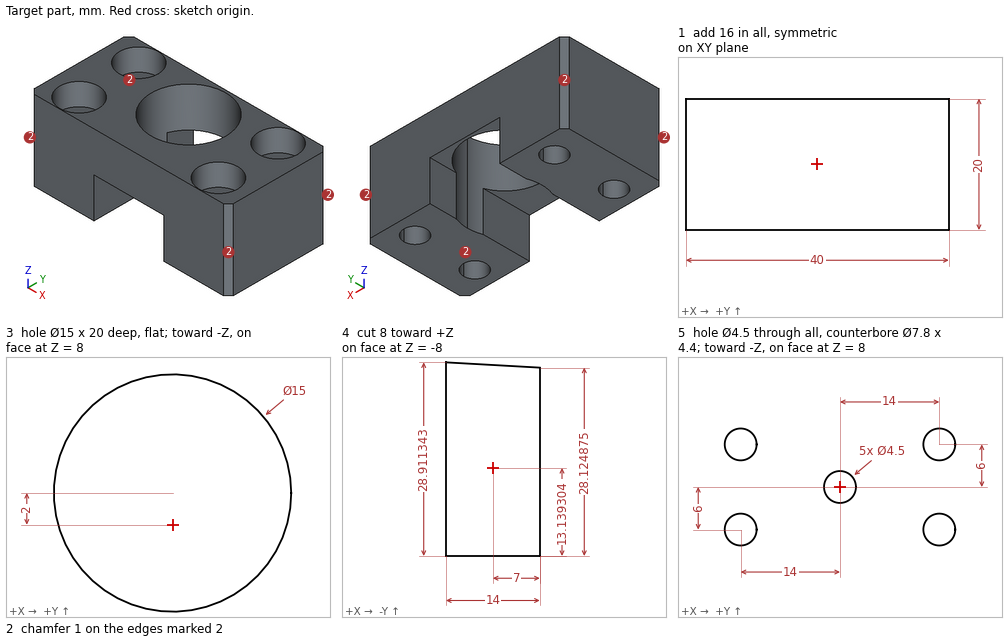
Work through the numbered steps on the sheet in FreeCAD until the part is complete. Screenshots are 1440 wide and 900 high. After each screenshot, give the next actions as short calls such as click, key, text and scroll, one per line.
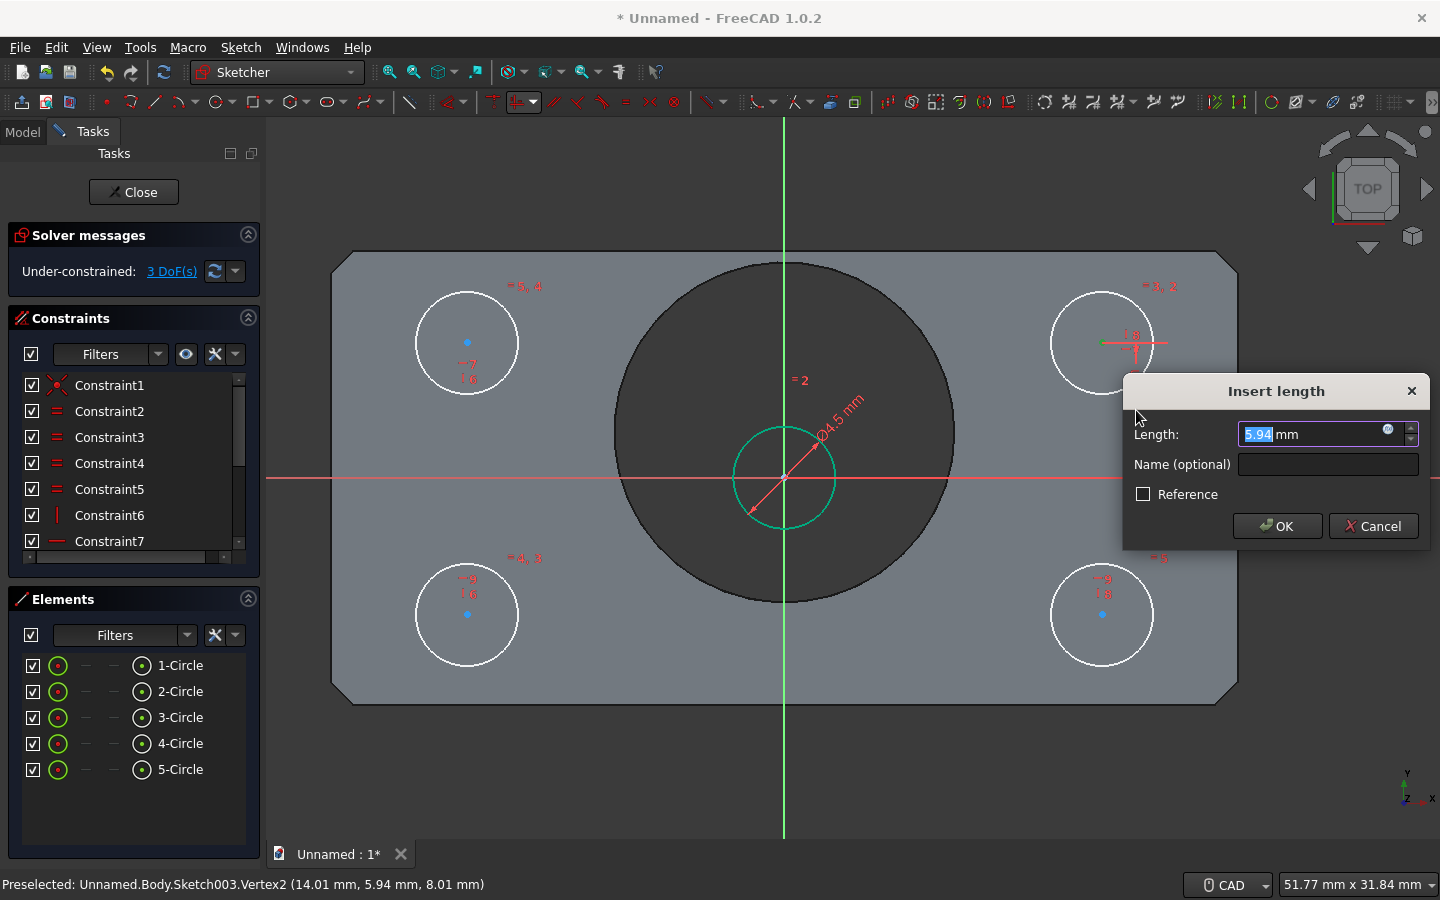
text(6)
key(Return)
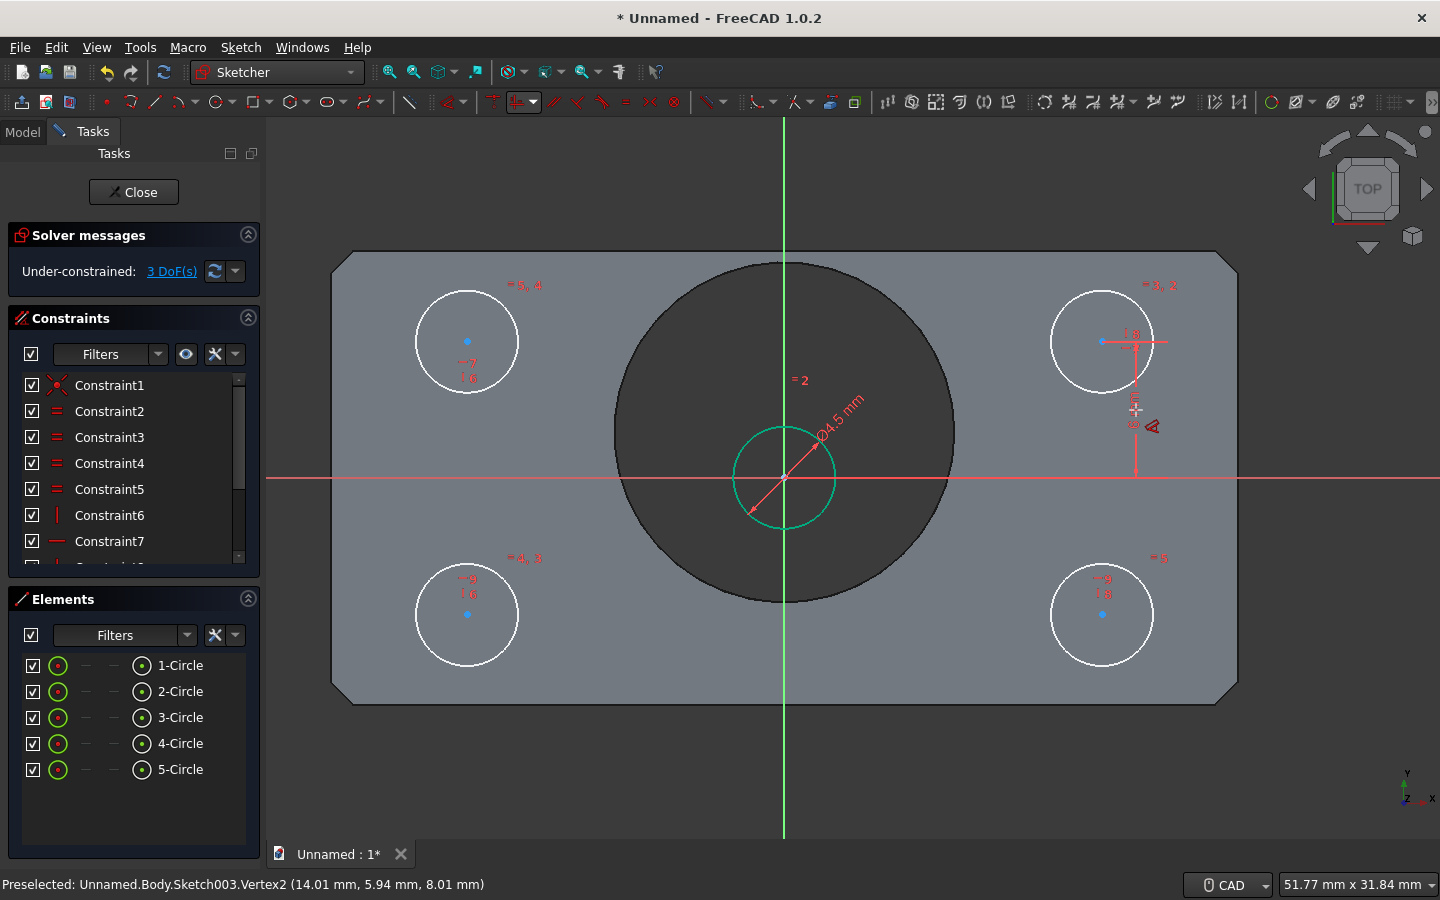
click(467, 615)
click(433, 546)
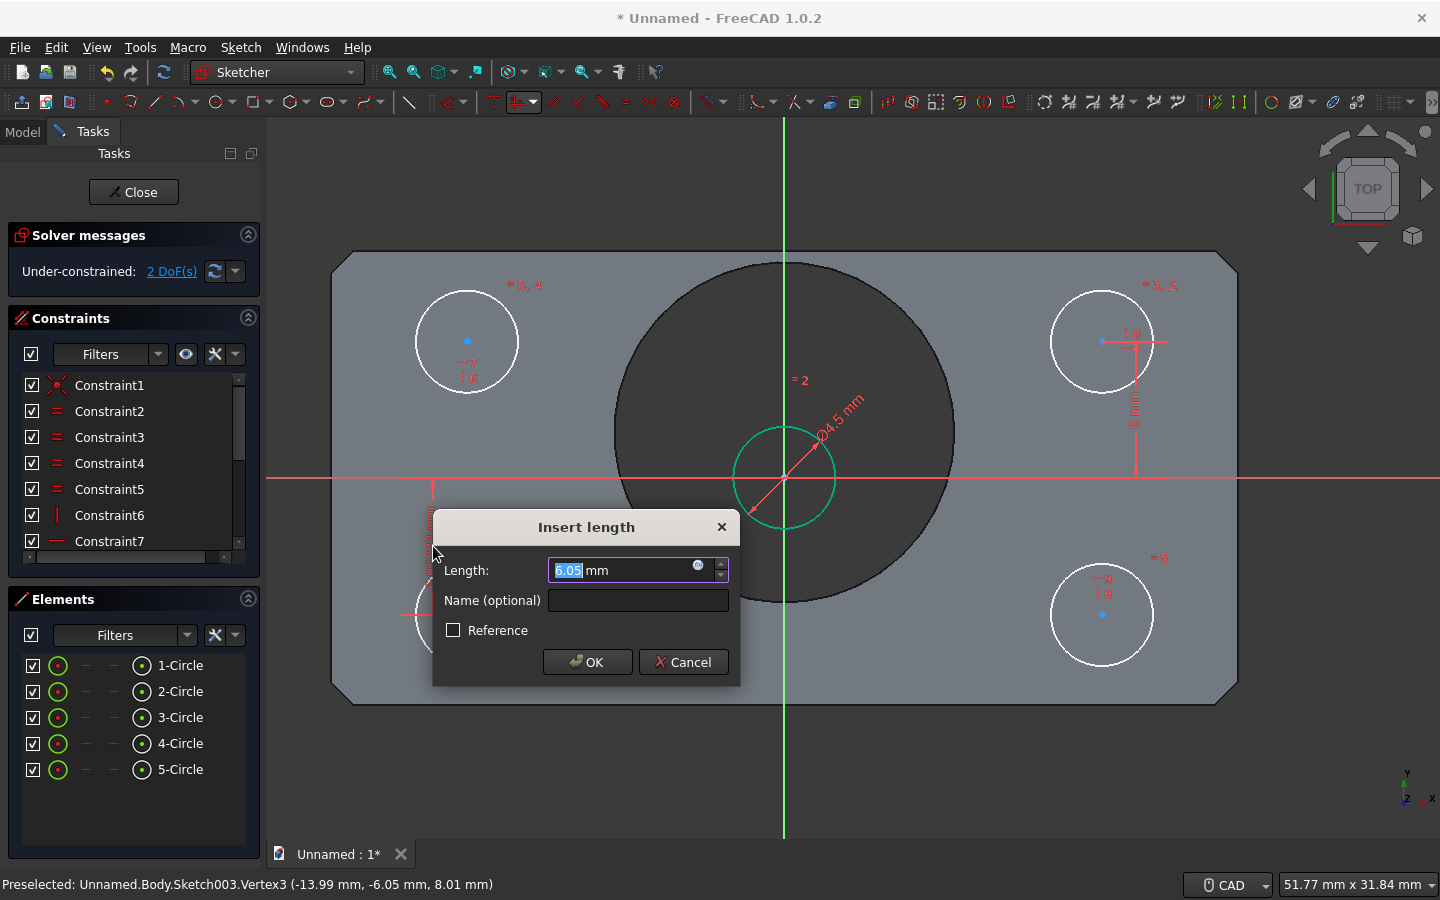
text(6)
key(Return)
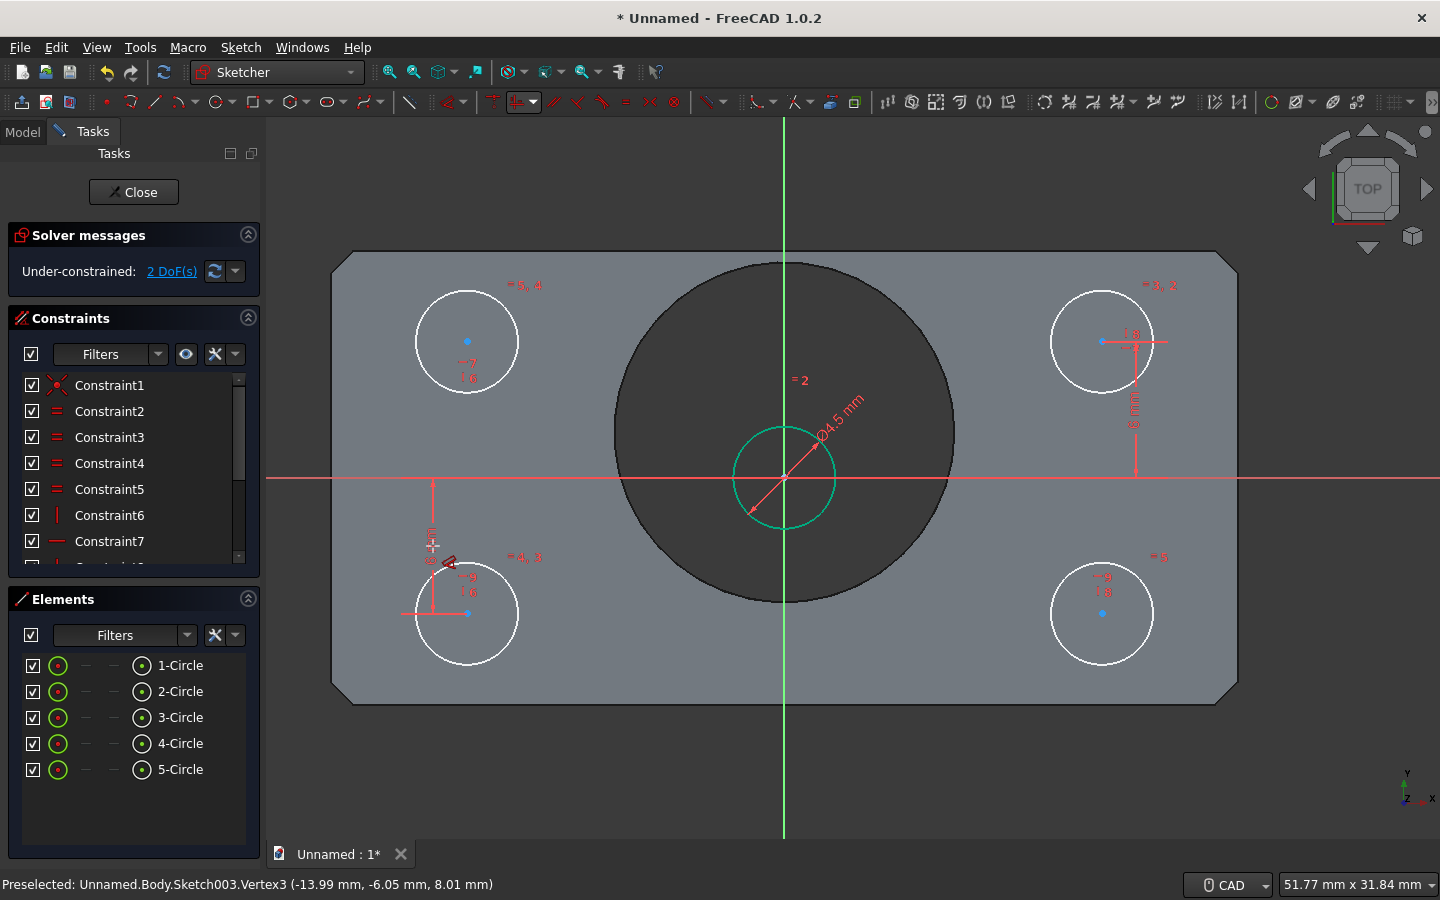
click(1102, 342)
click(943, 308)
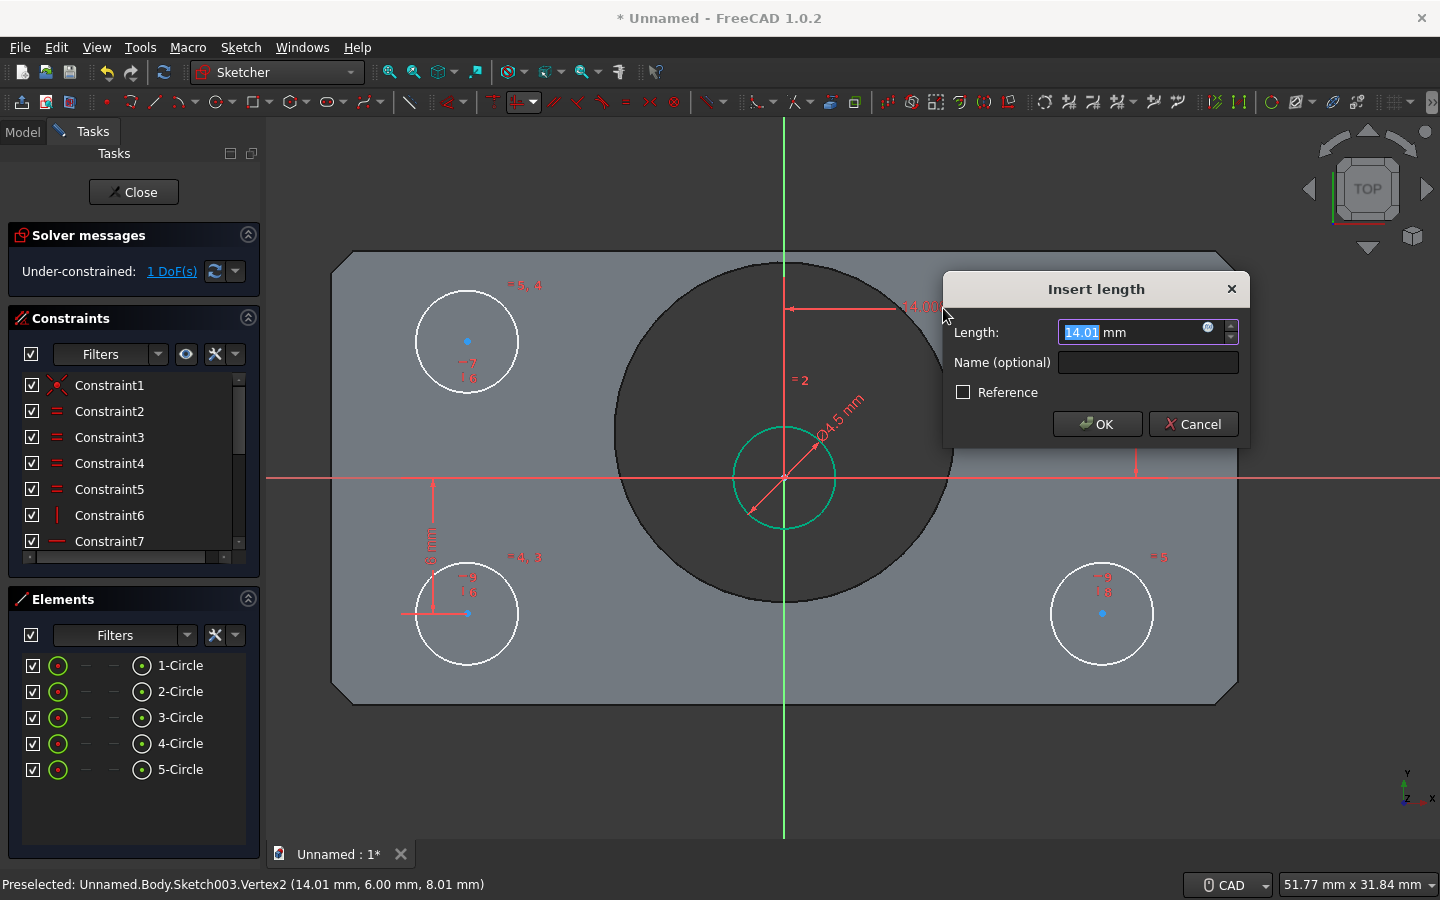
text(14)
key(Return)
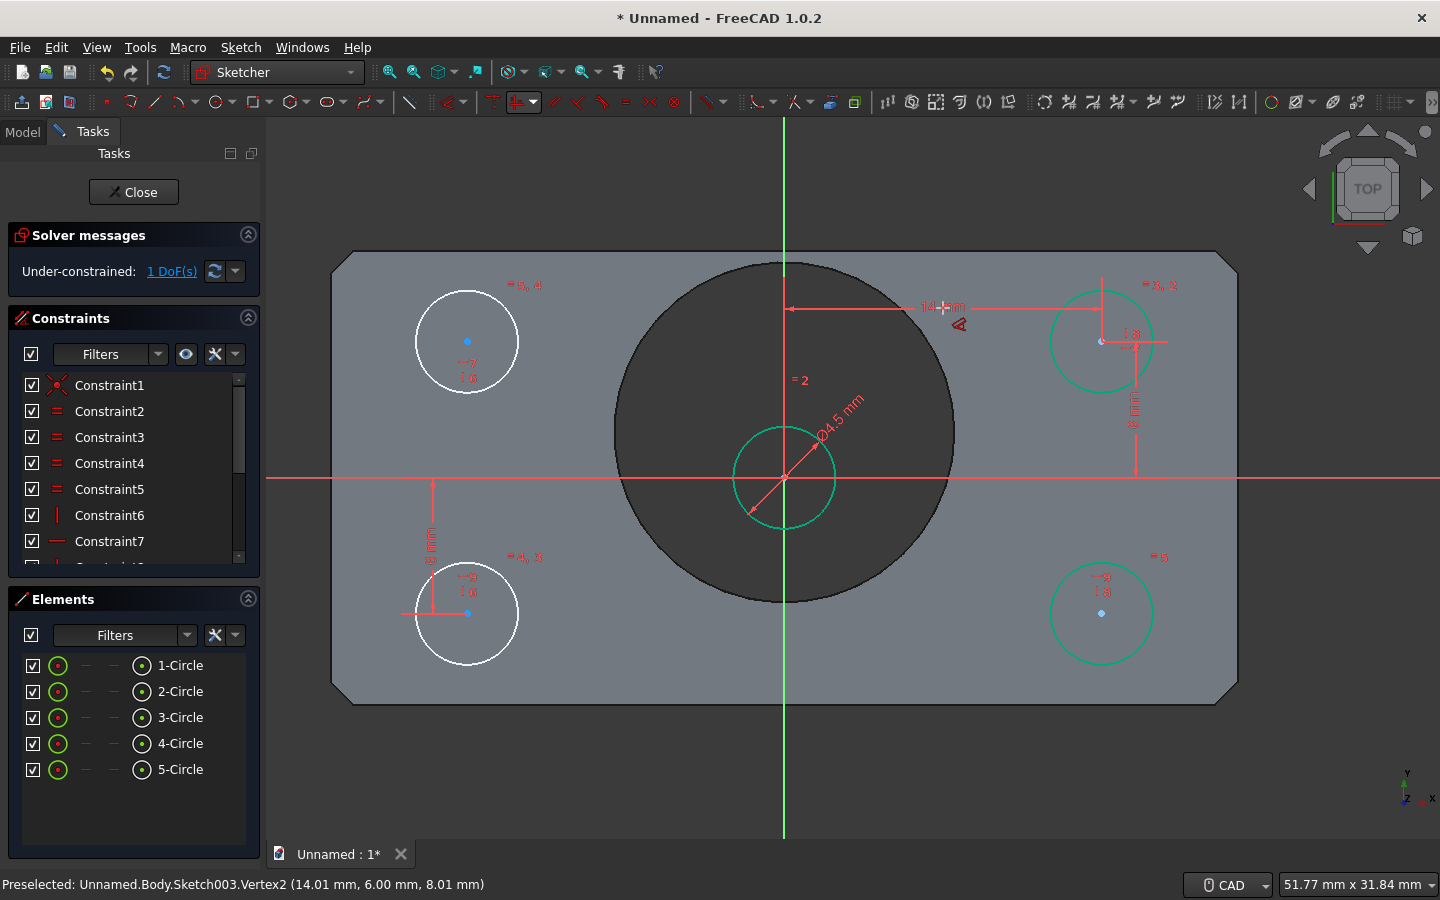
click(467, 614)
click(626, 648)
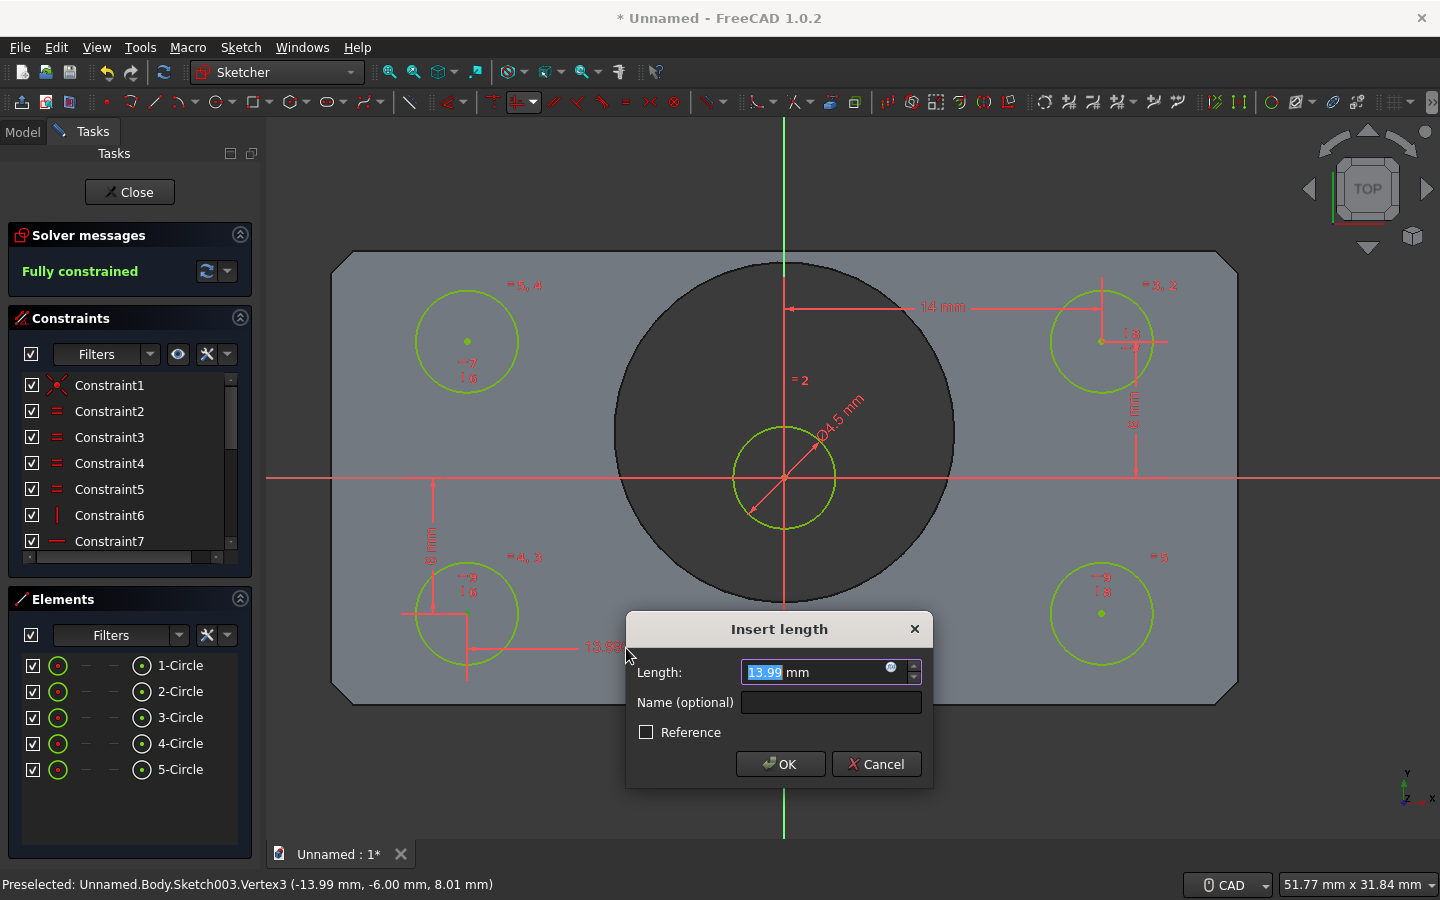
text(14)
key(Return)
key(Escape)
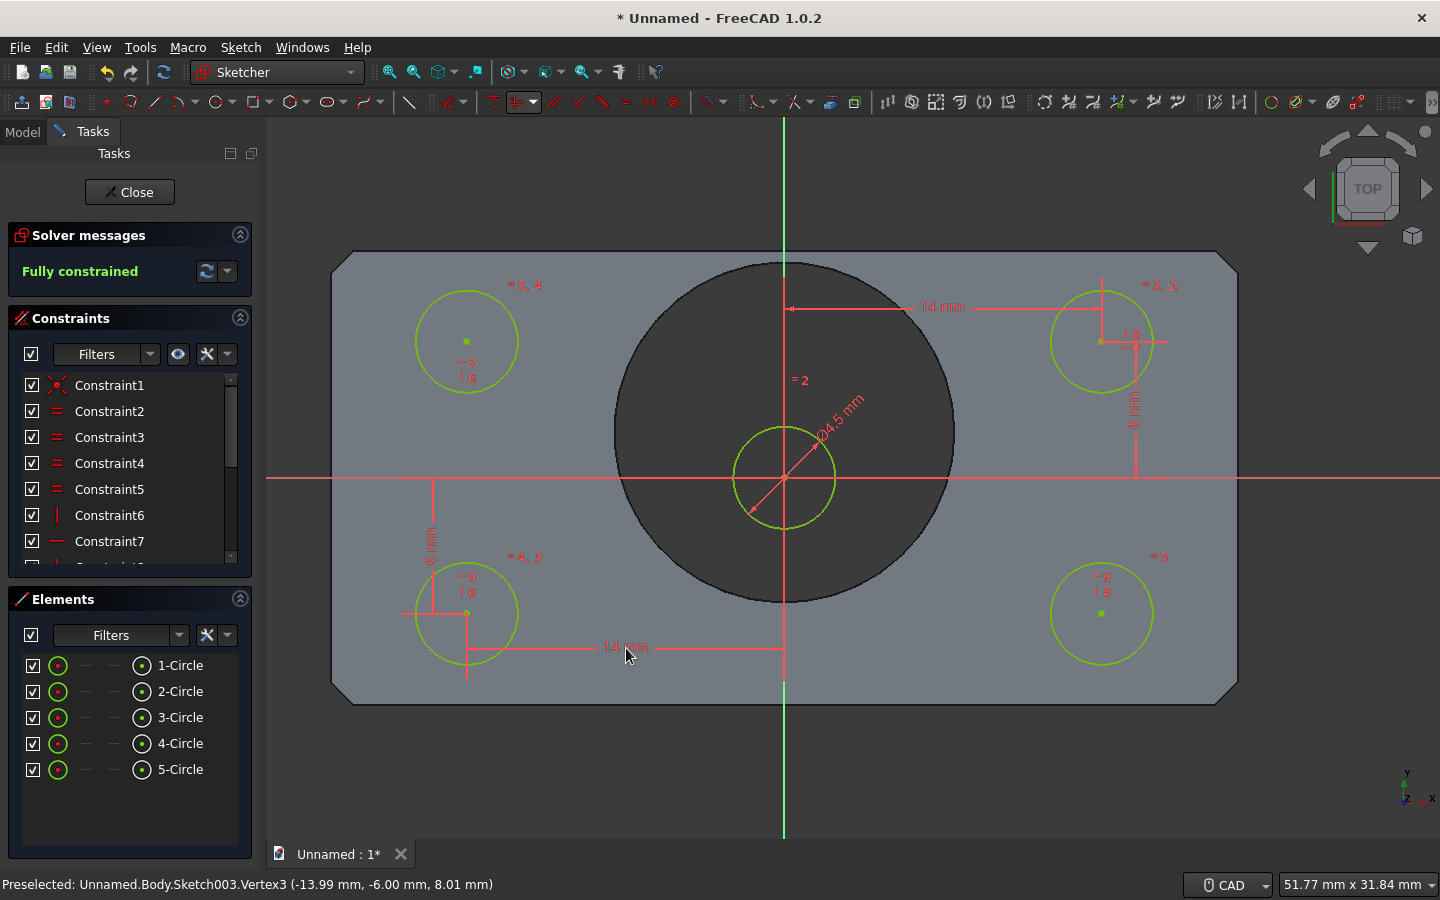
click(130, 192)